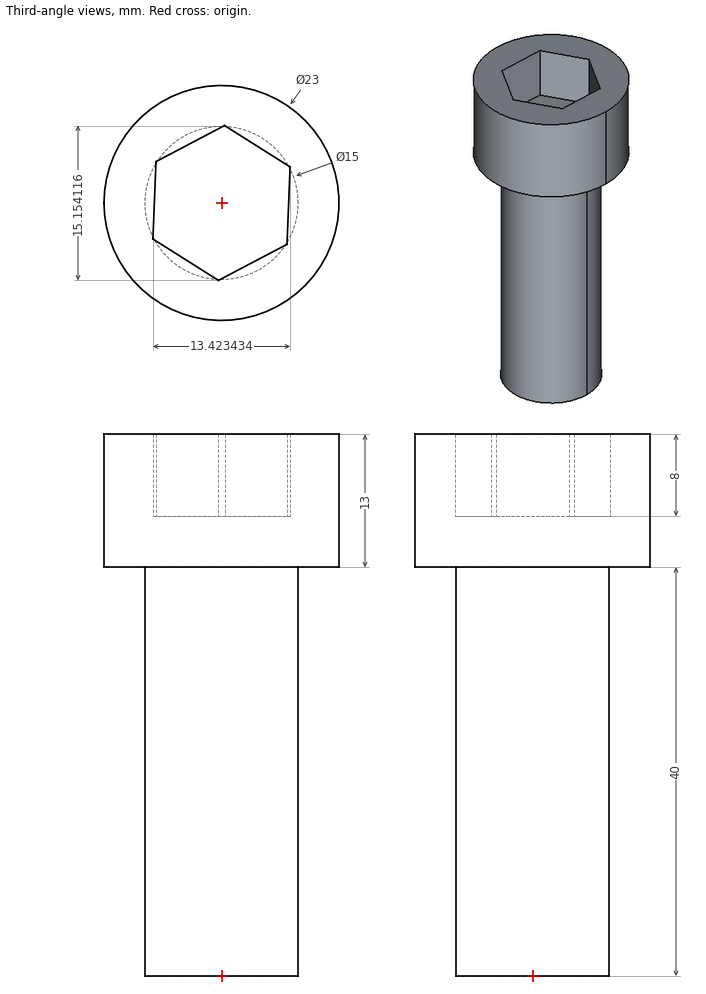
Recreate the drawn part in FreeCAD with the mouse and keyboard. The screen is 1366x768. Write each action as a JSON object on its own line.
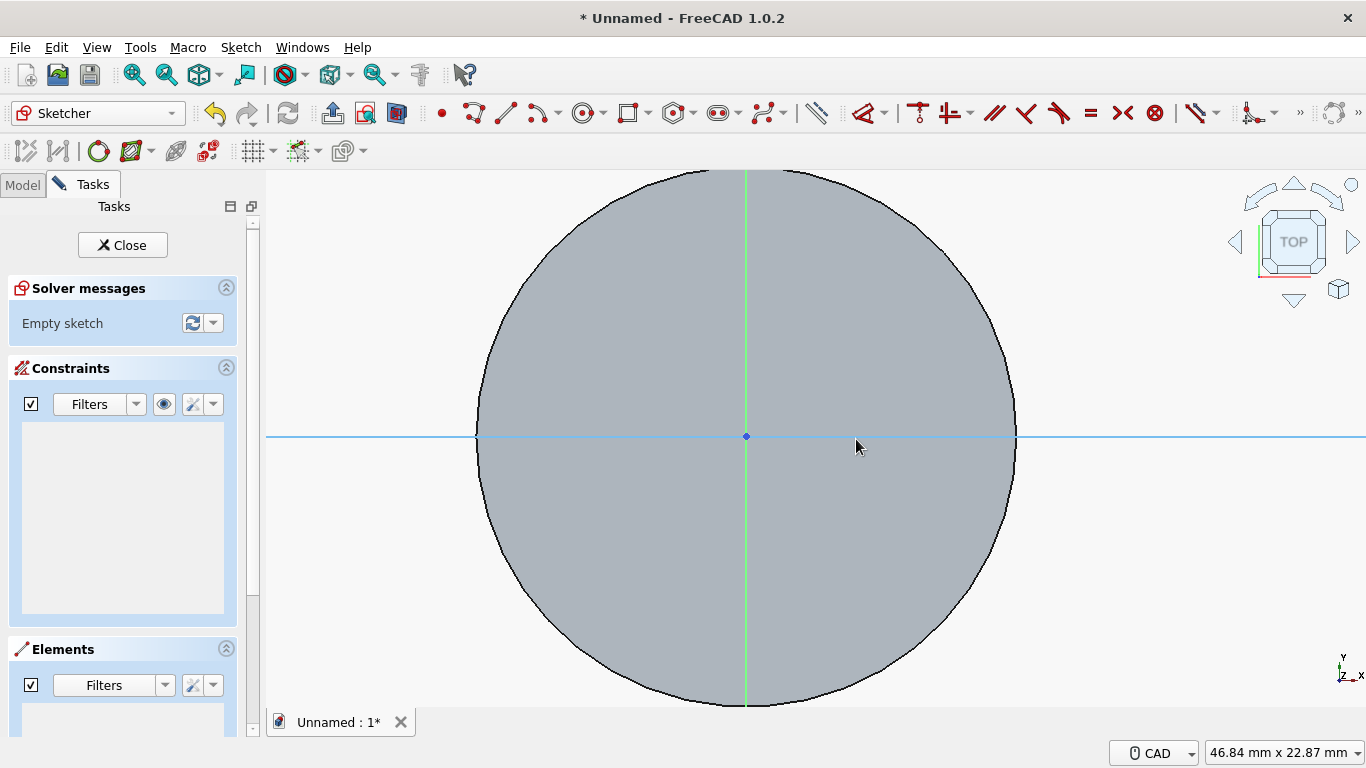
{"action": "left_click", "coordinate": [674, 114]}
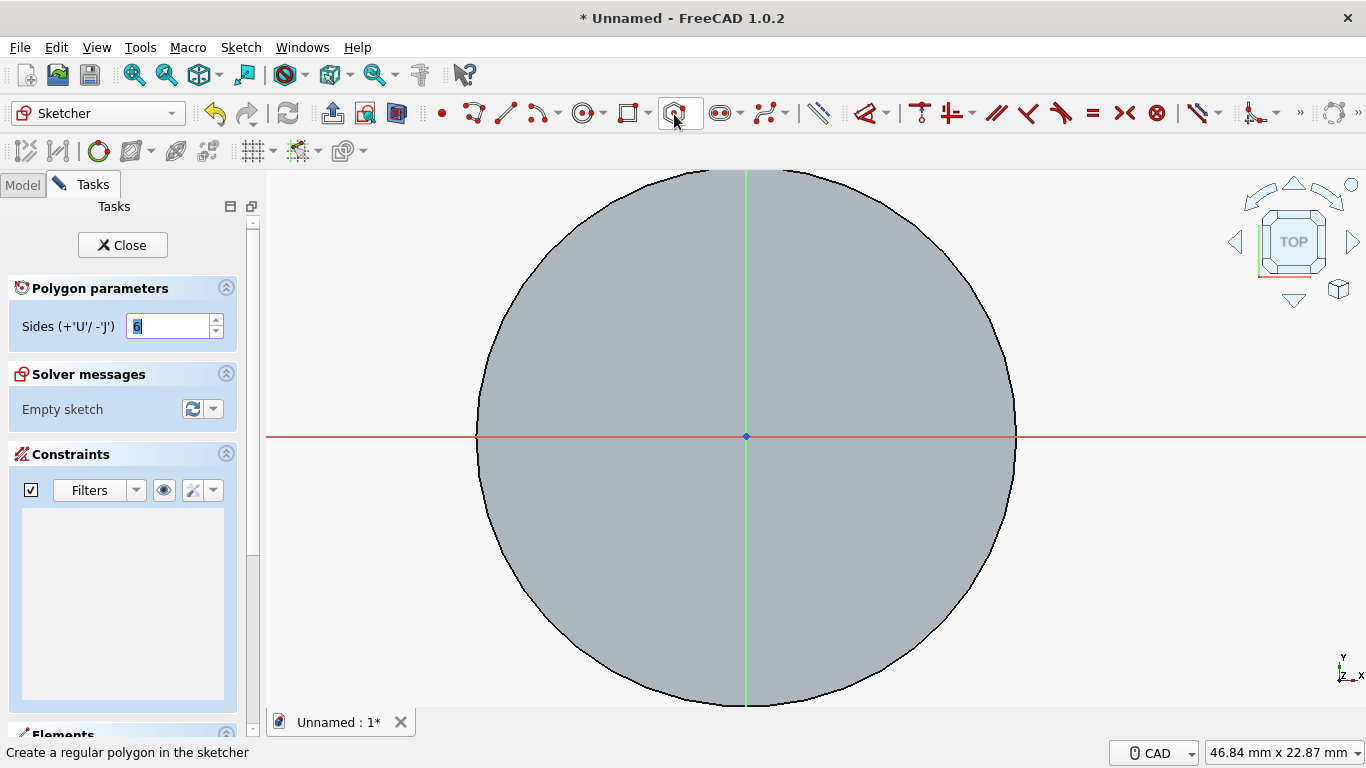
{"action": "left_click", "coordinate": [746, 437]}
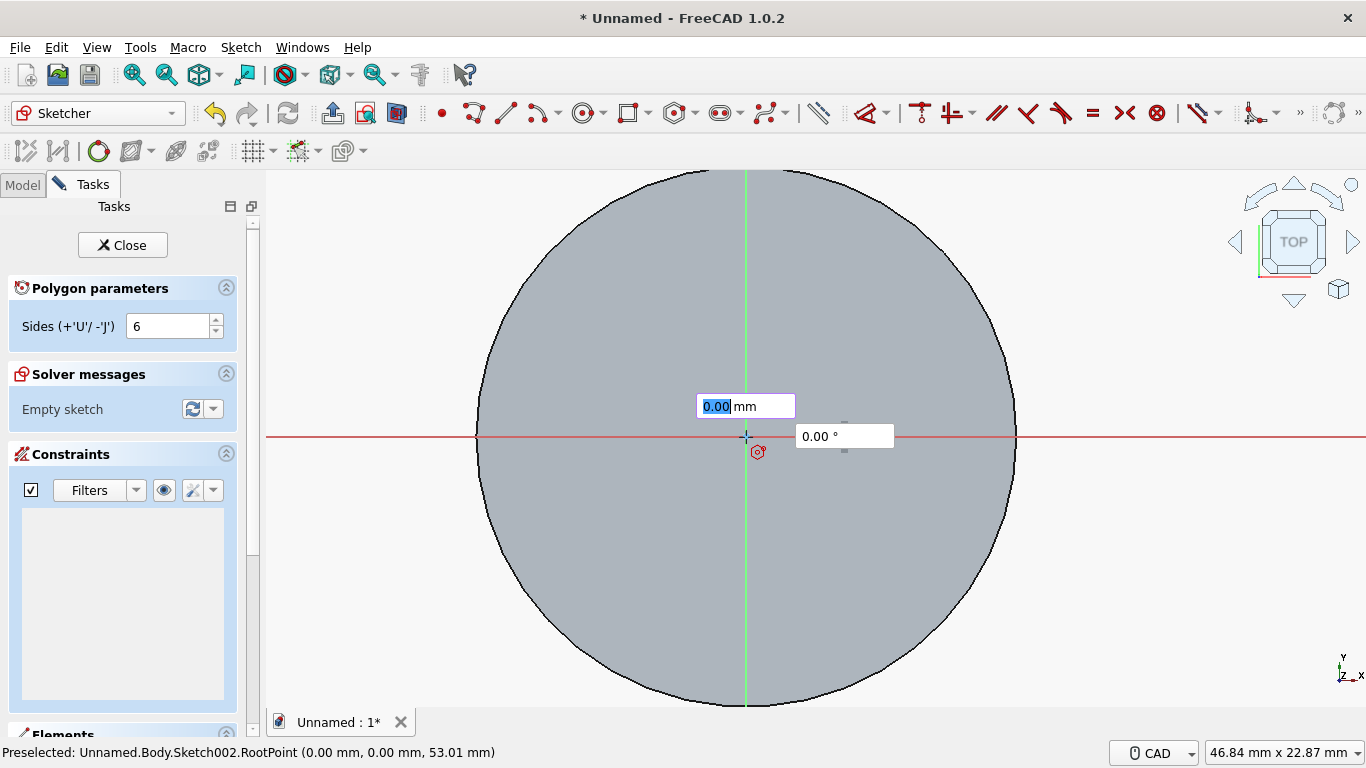
{"action": "left_click", "coordinate": [897, 532]}
{"action": "right_click", "coordinate": [897, 532]}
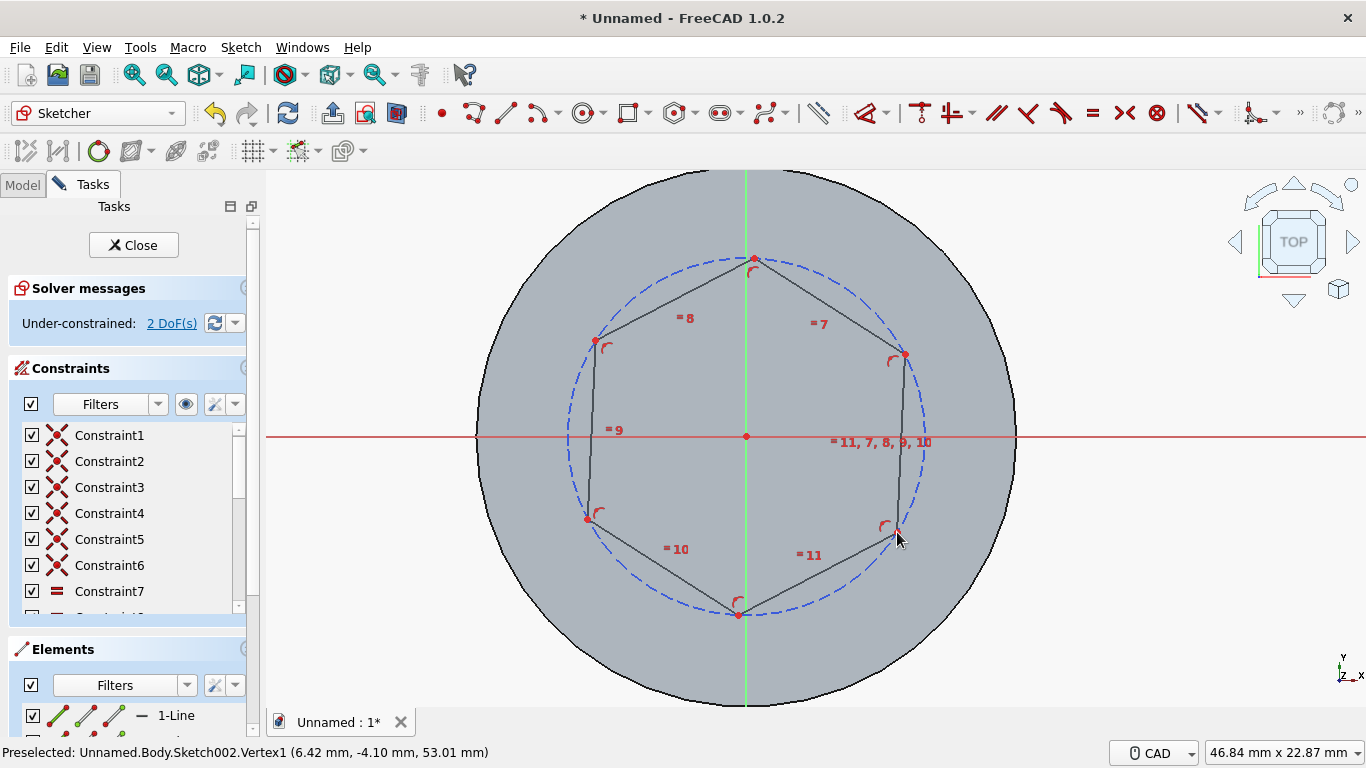
{"action": "left_click", "coordinate": [866, 114]}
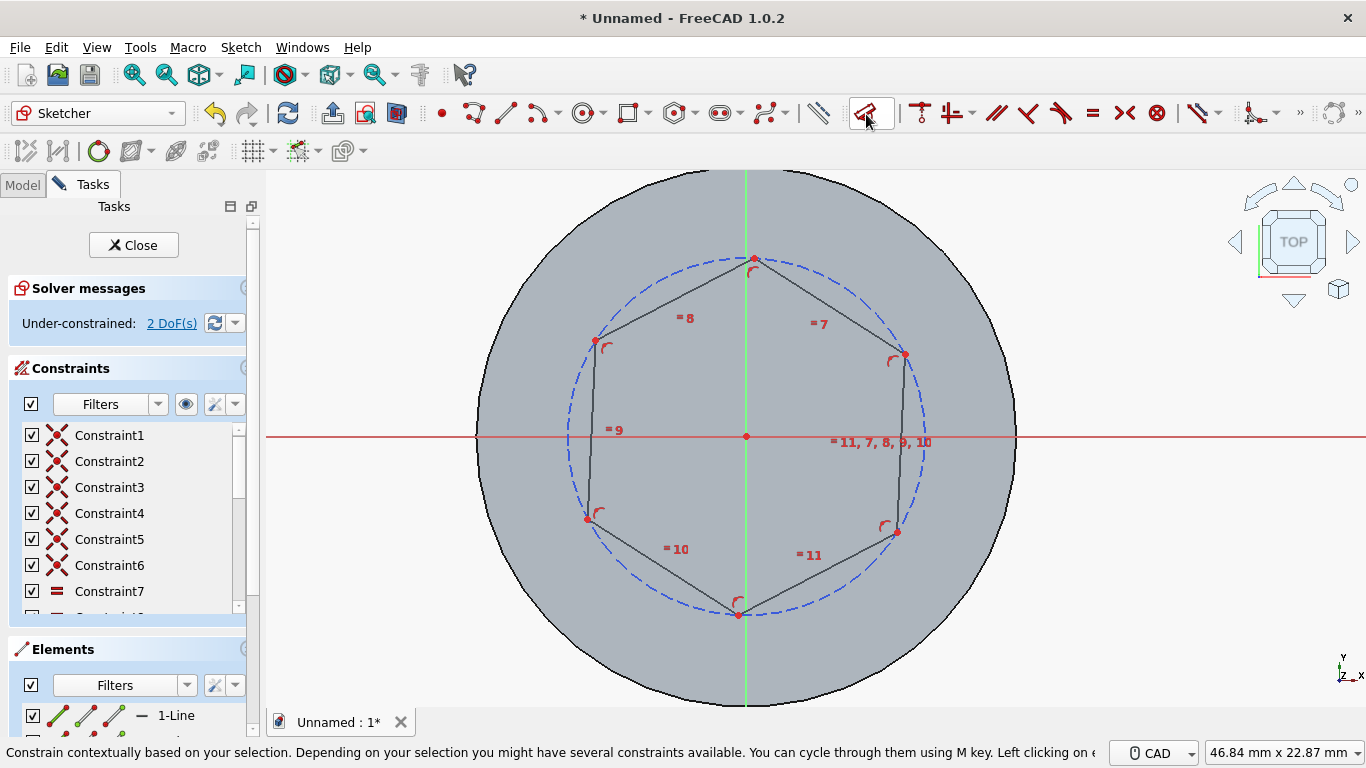
{"action": "left_click", "coordinate": [588, 519]}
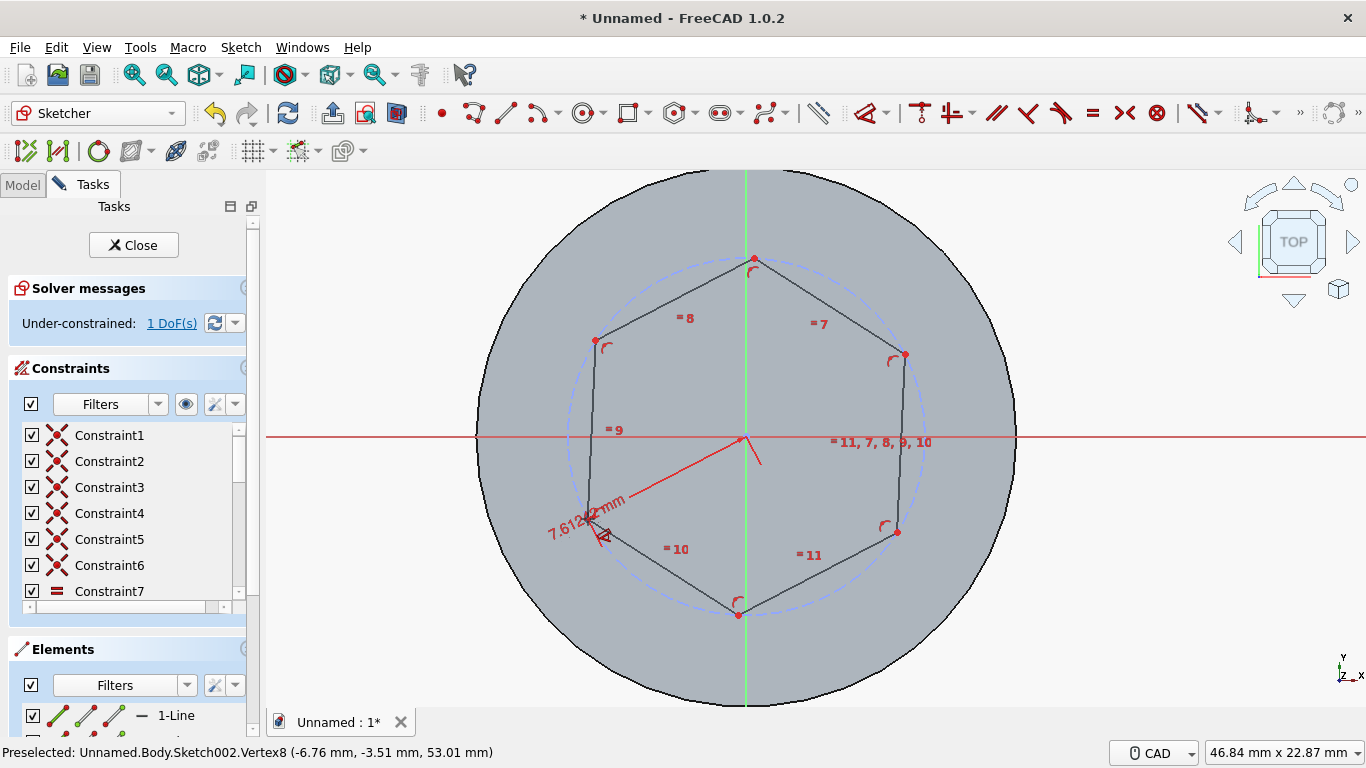
{"action": "left_click", "coordinate": [905, 354]}
{"action": "left_click", "coordinate": [673, 553]}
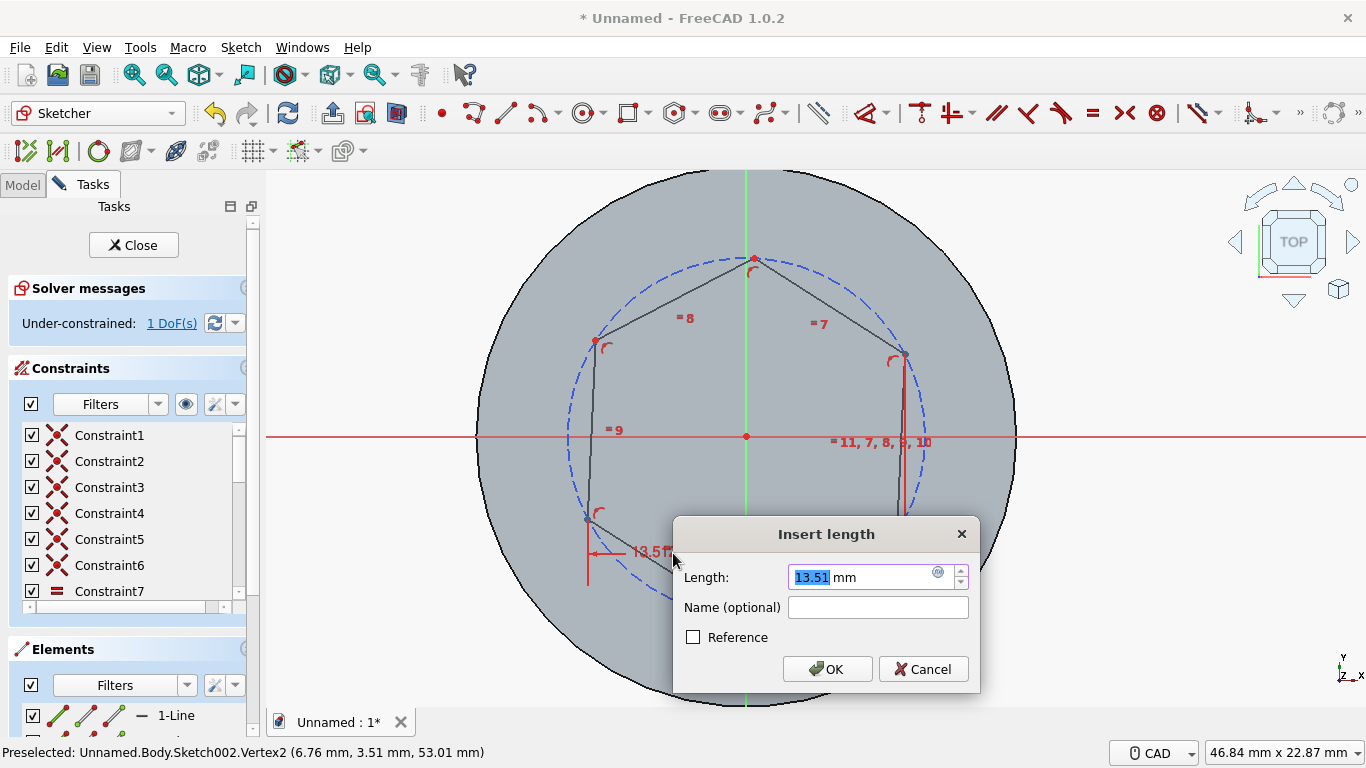
{"action": "type", "text": "13.423434"}
{"action": "key", "text": "Return"}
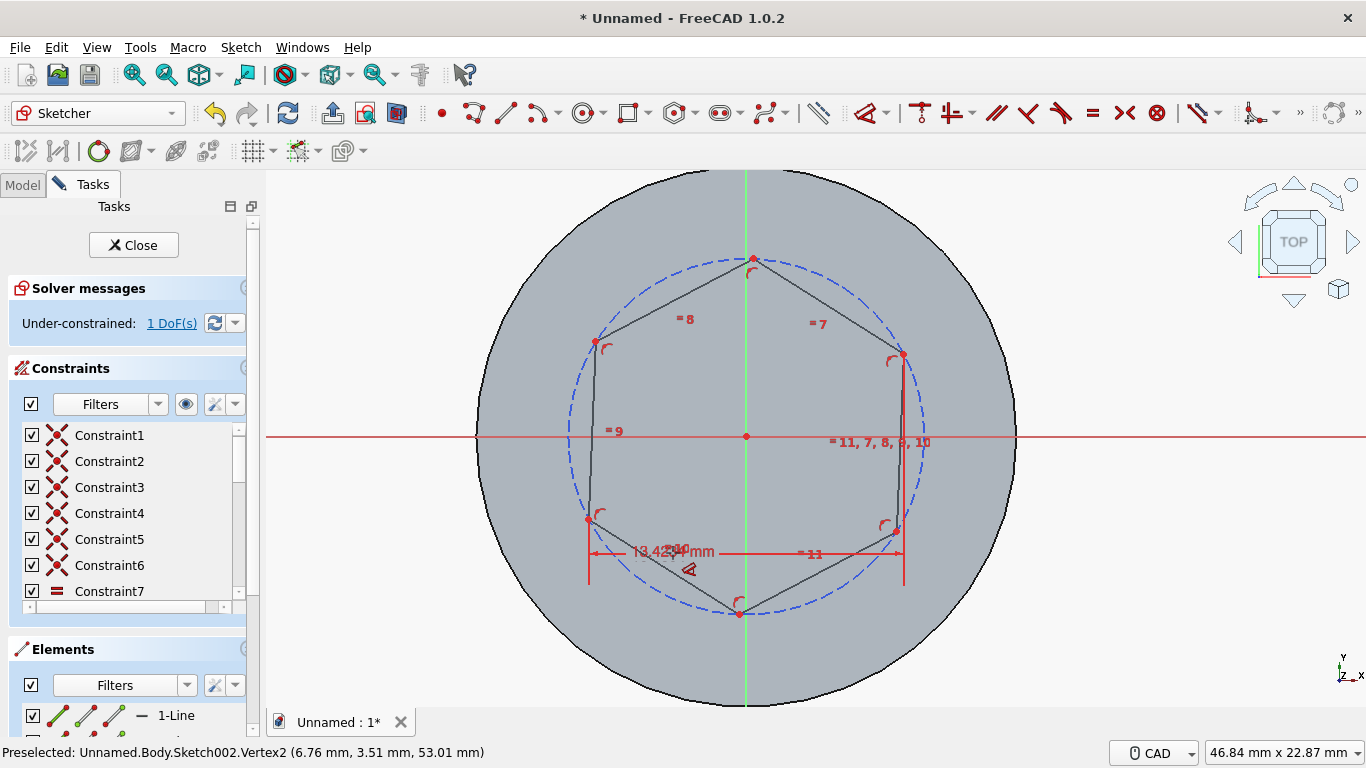
{"action": "left_click", "coordinate": [739, 615]}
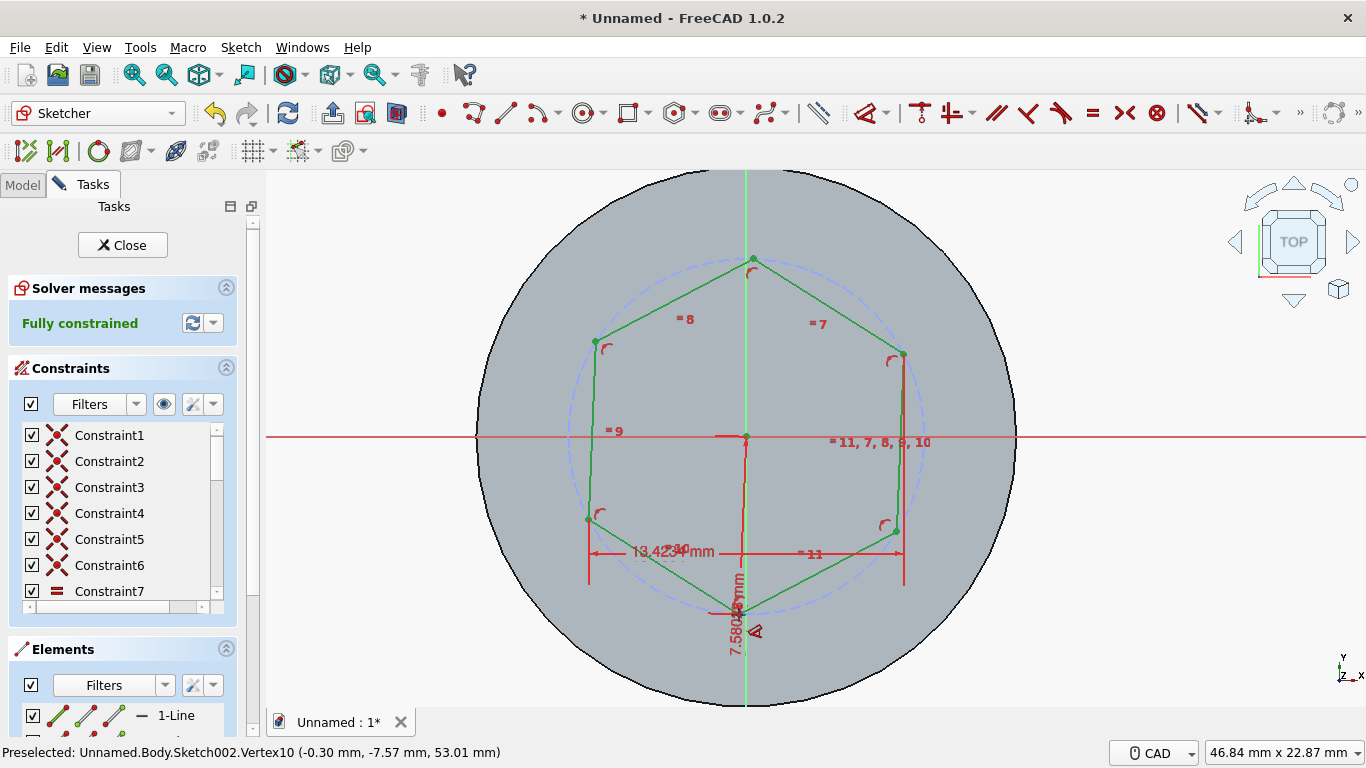
{"action": "left_click", "coordinate": [753, 259]}
{"action": "left_click", "coordinate": [787, 355]}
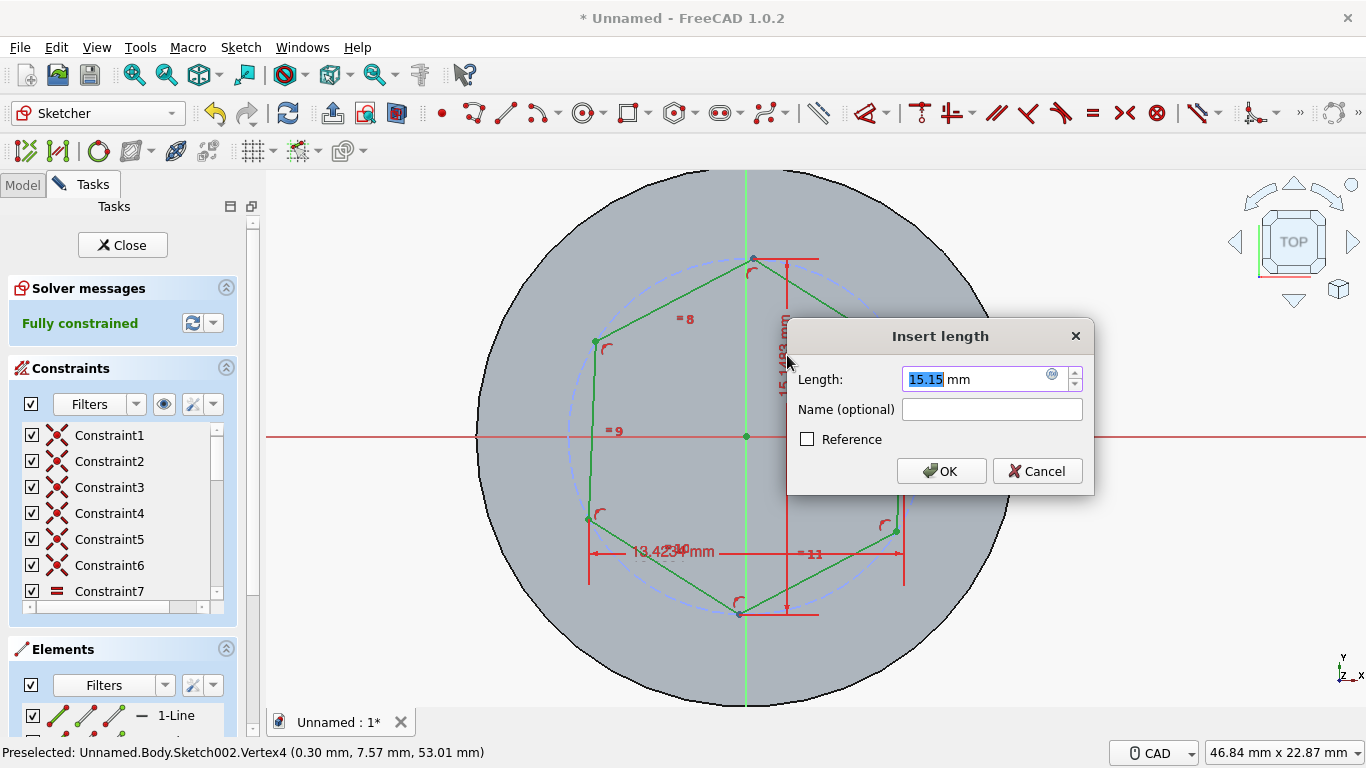
{"action": "type", "text": "15.154116"}
{"action": "key", "text": "Return"}
{"action": "key", "text": "Escape"}